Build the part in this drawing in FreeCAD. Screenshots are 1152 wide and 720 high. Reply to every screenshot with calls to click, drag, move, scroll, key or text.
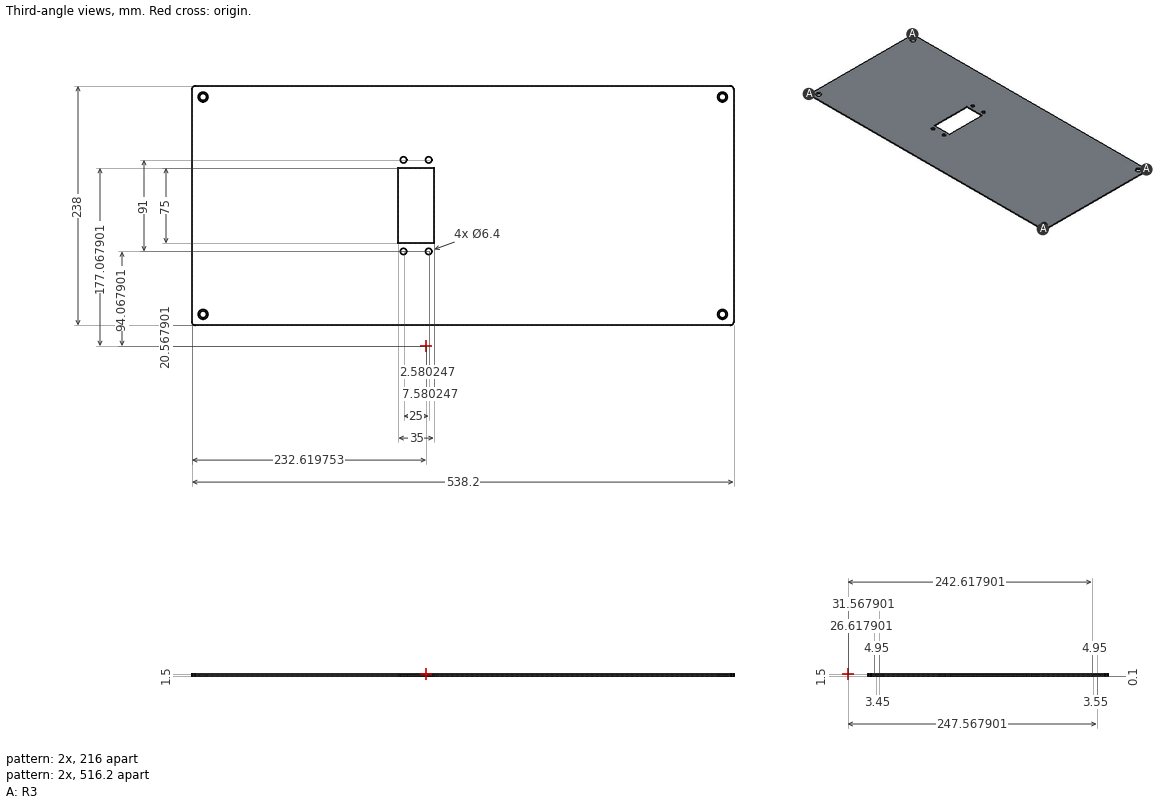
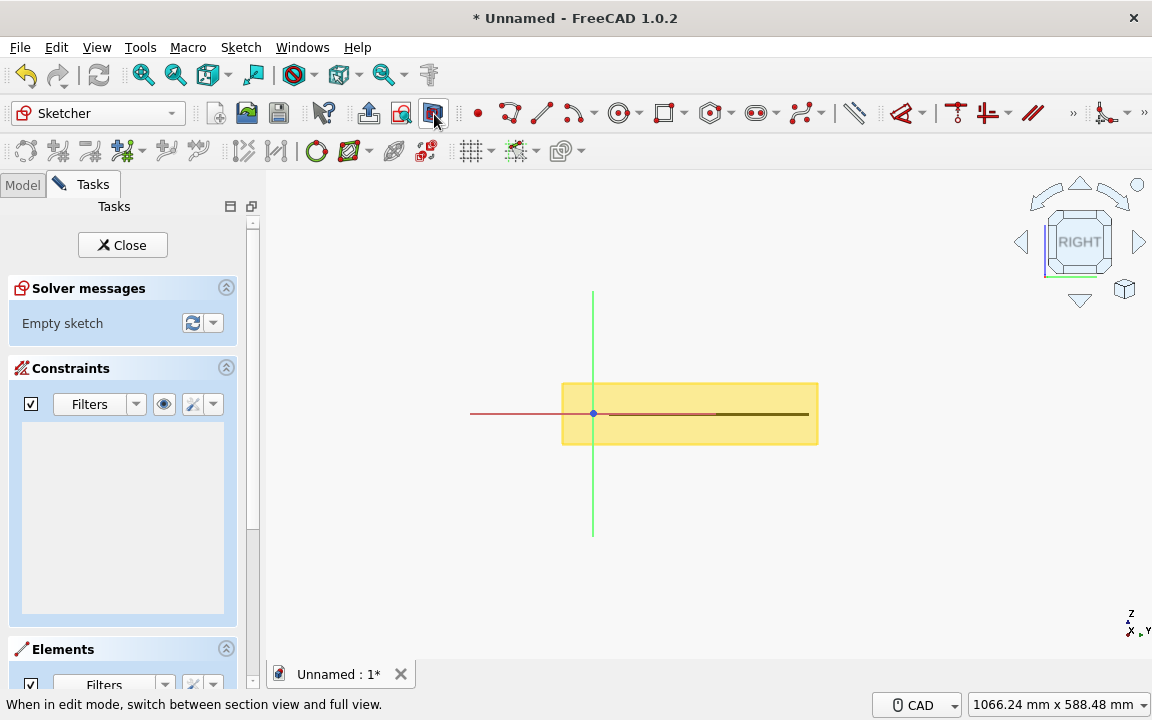
scroll(805, 415, up, 15)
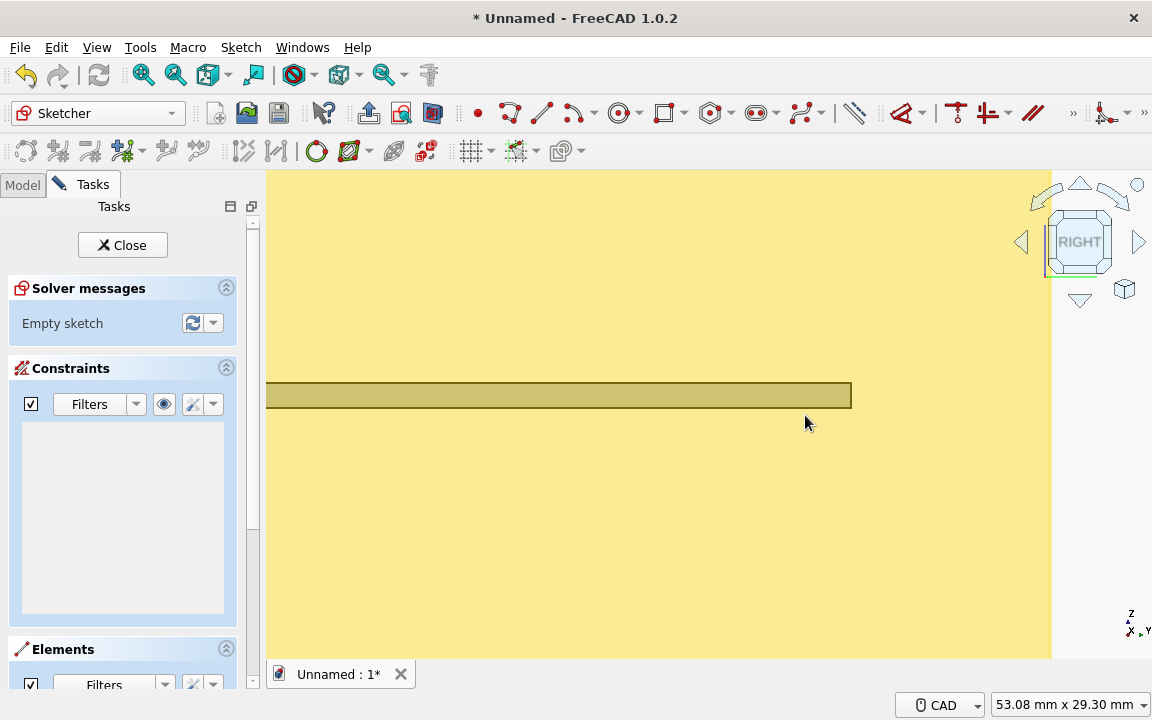
scroll(624, 400, up, 9)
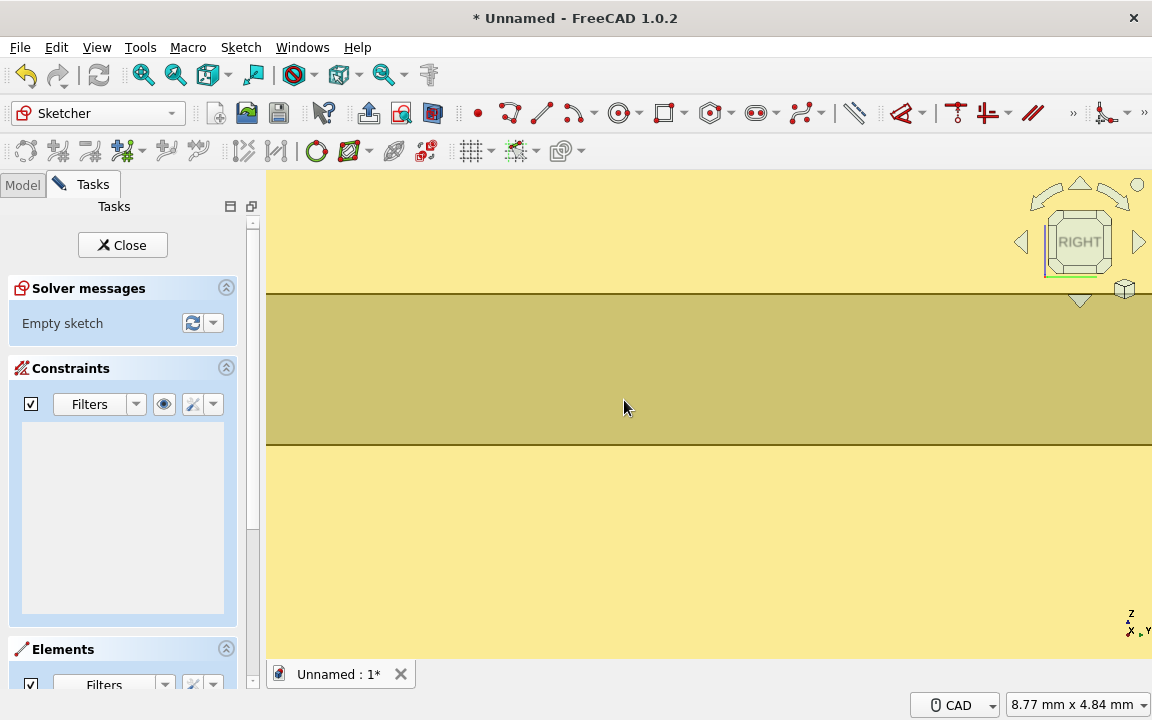
click(510, 114)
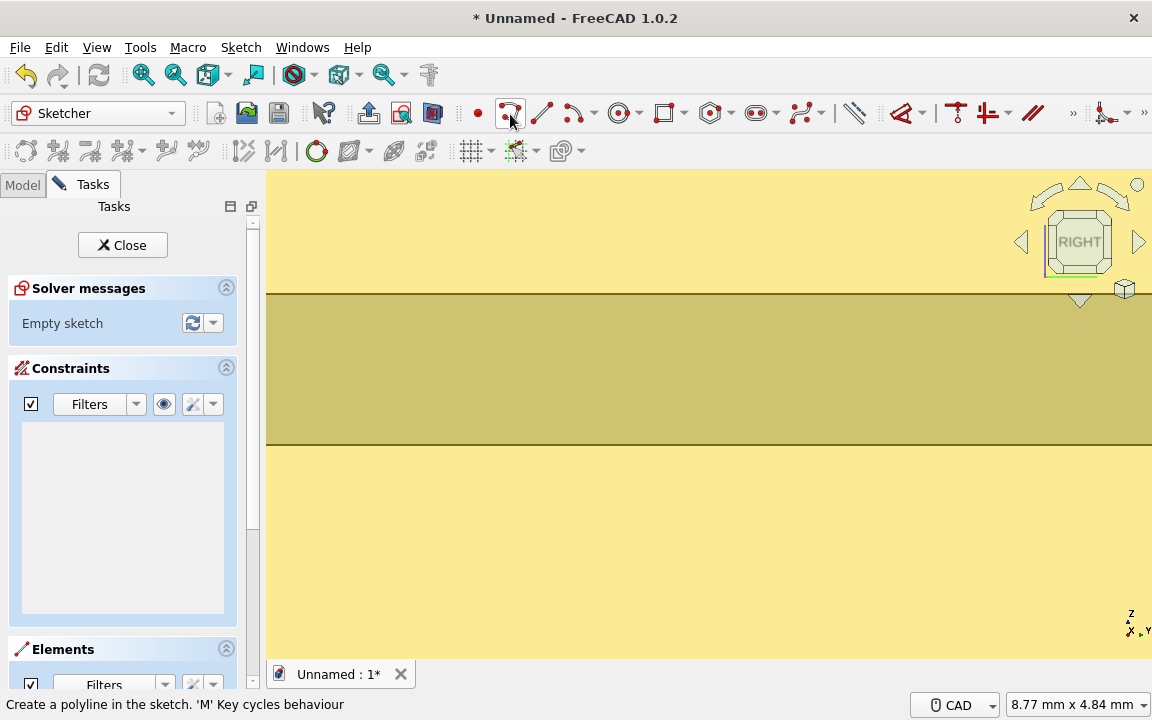
click(387, 294)
click(528, 435)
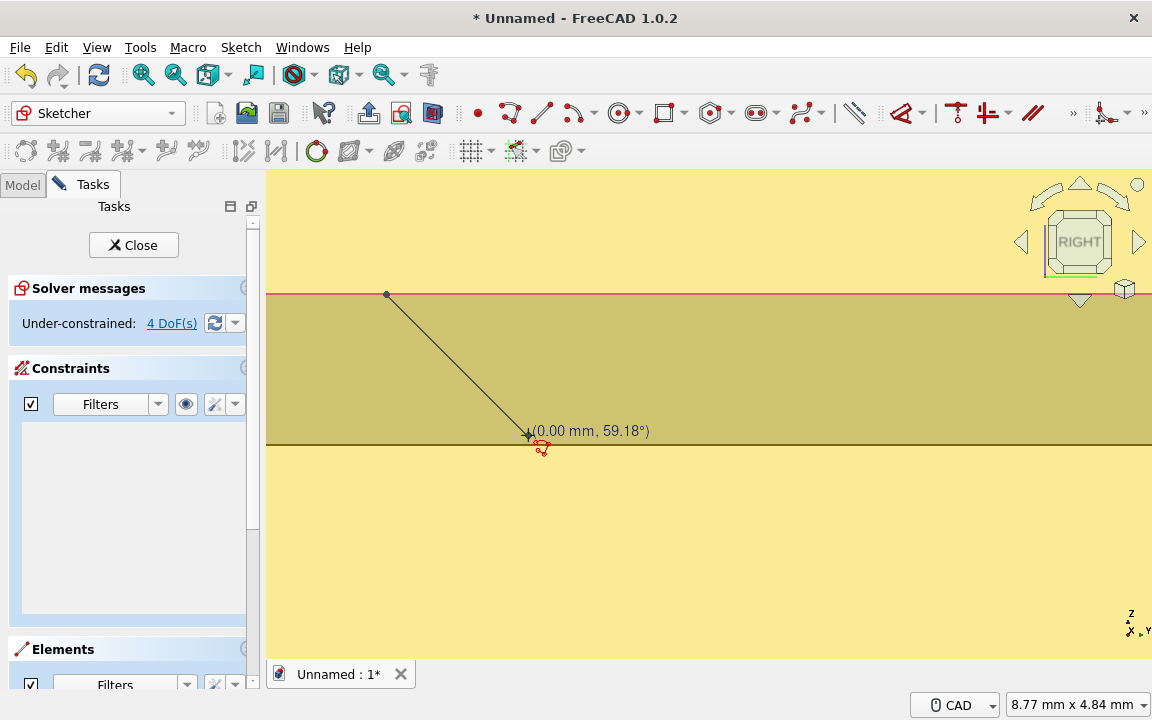
scroll(528, 445, up, 3)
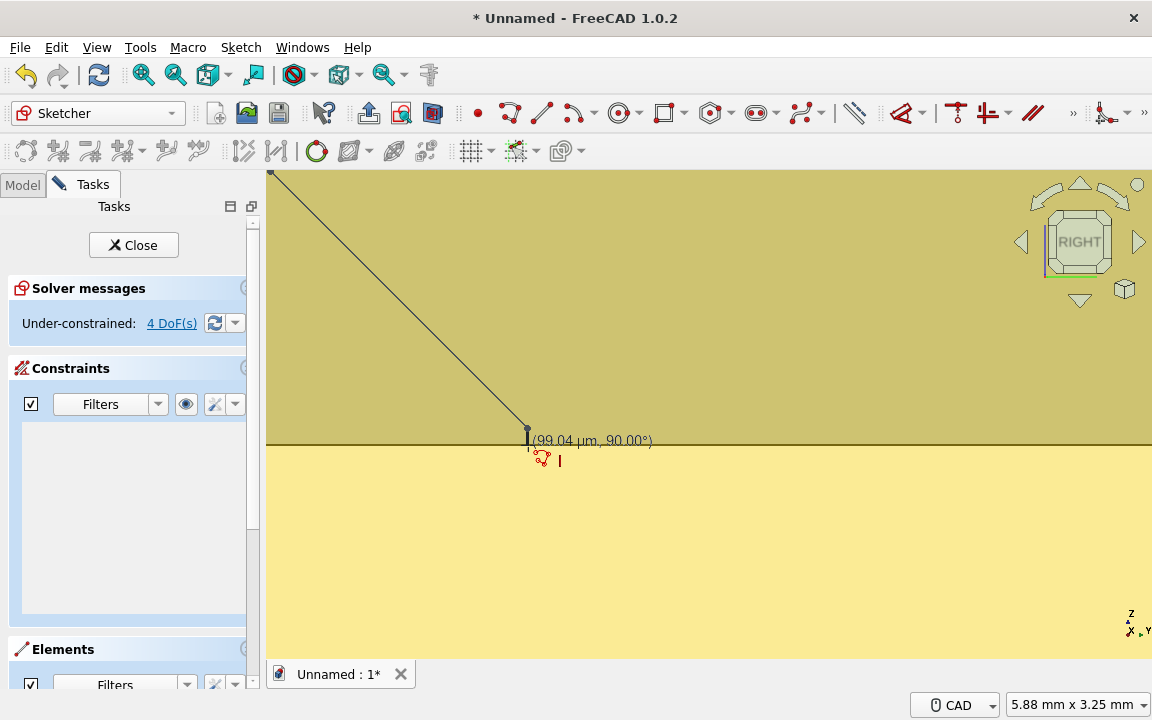
click(528, 445)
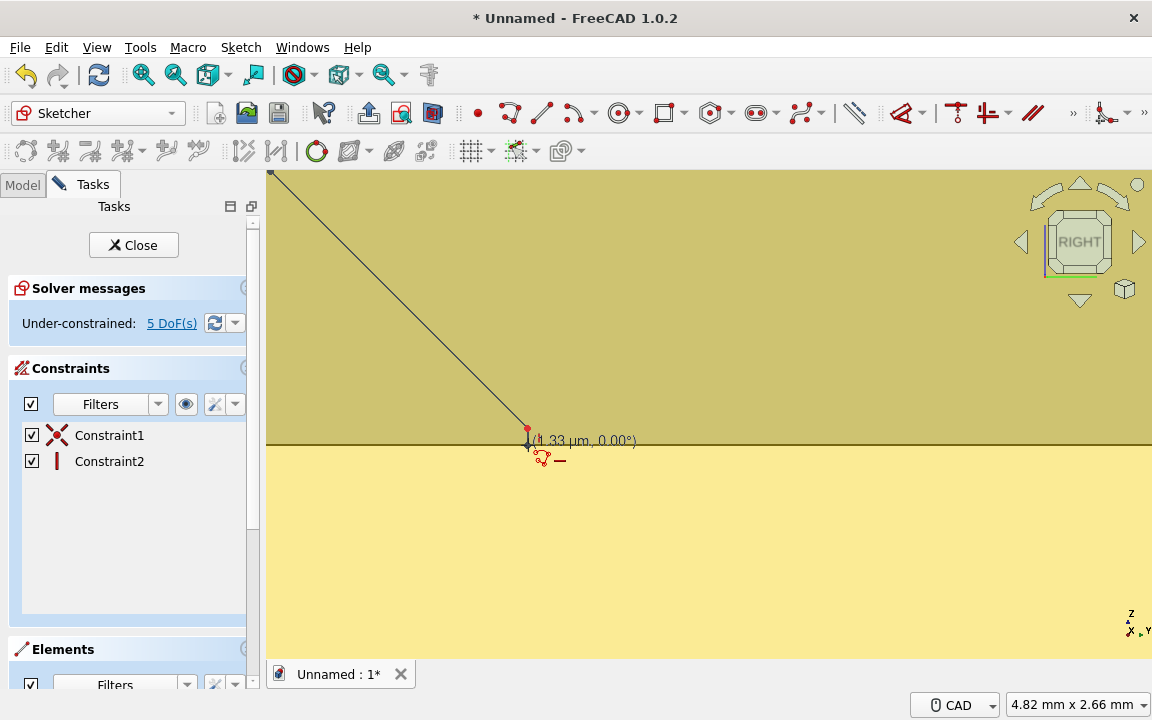
scroll(537, 456, down, 3)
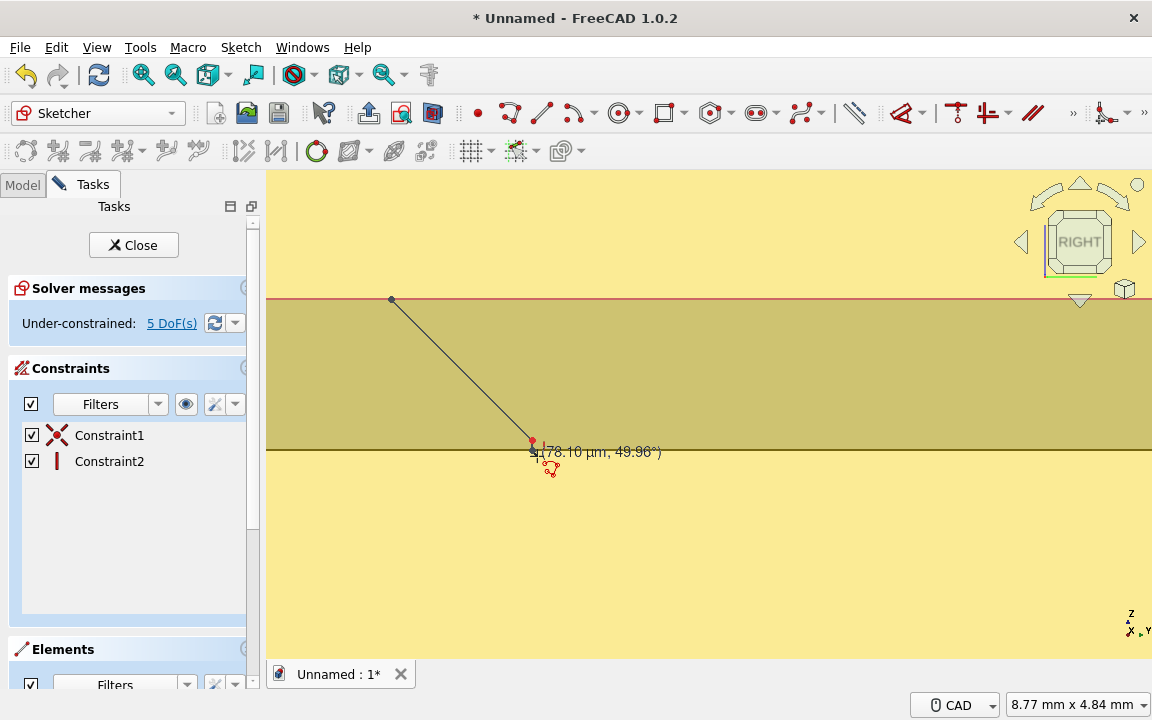
click(890, 450)
click(890, 308)
click(391, 300)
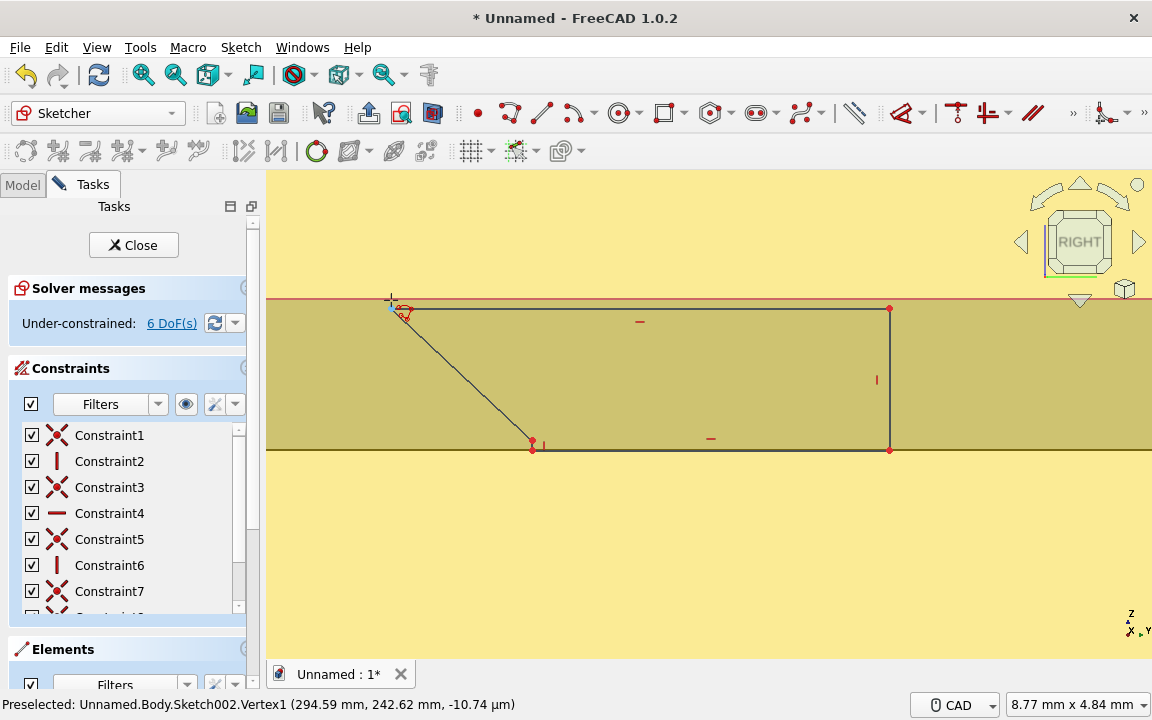
click(542, 114)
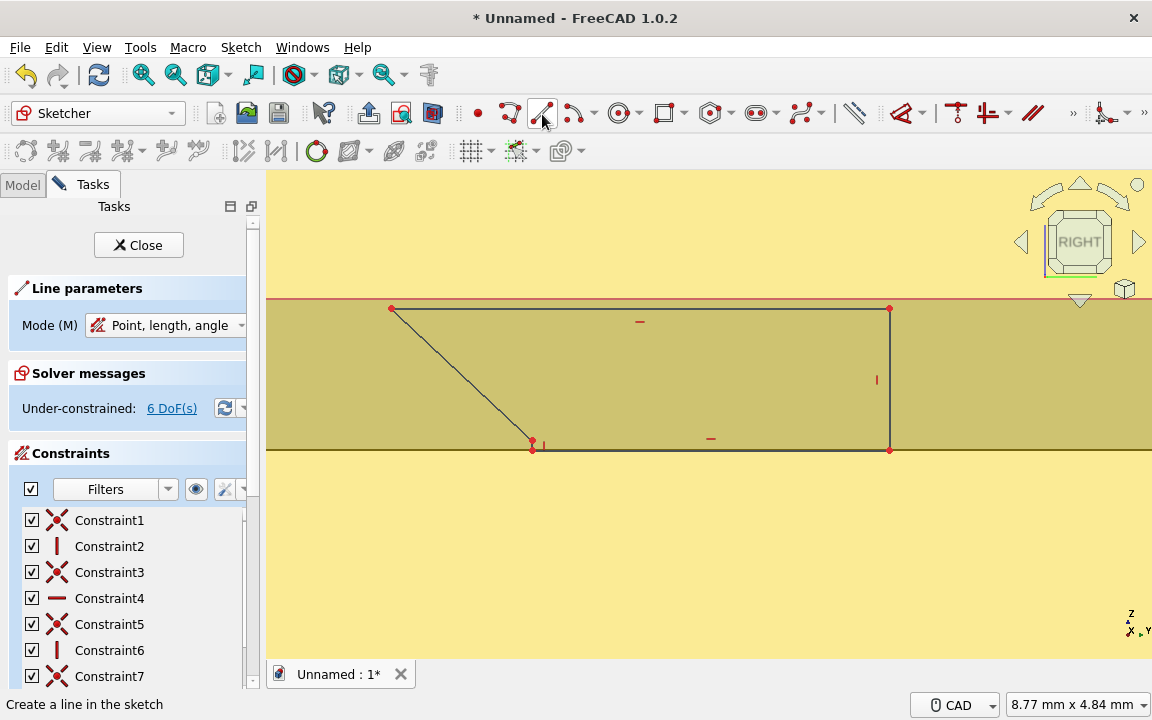
click(890, 470)
click(890, 530)
key(Escape)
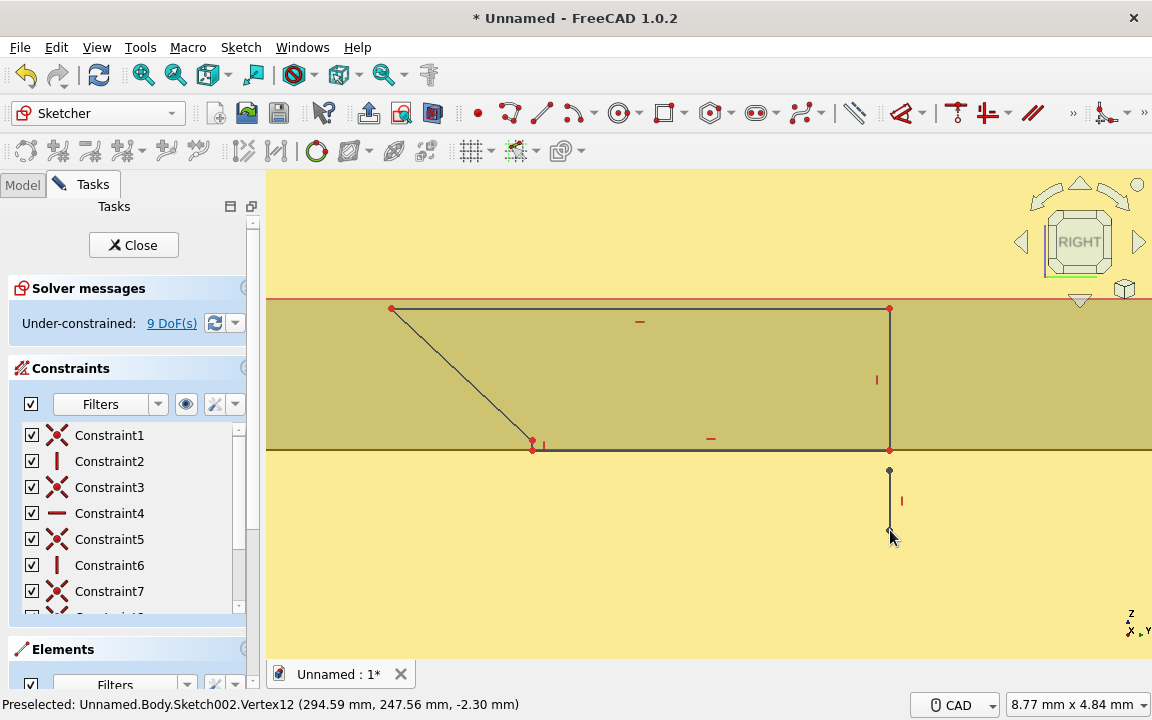
click(890, 489)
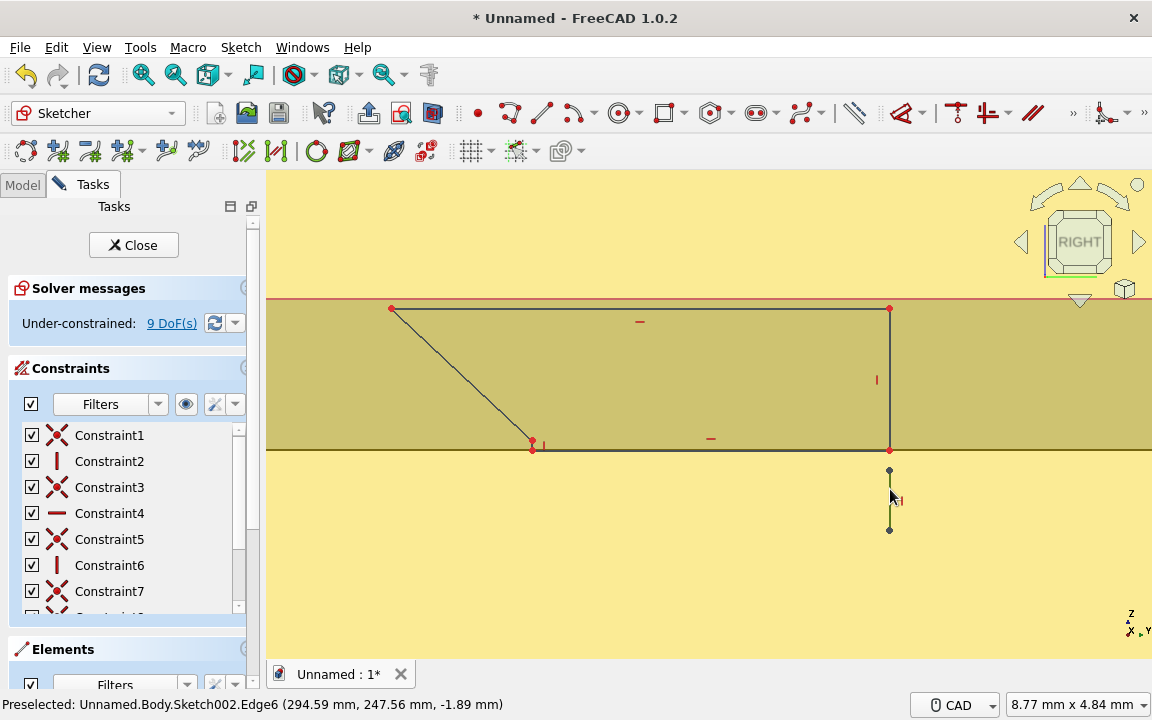
click(856, 114)